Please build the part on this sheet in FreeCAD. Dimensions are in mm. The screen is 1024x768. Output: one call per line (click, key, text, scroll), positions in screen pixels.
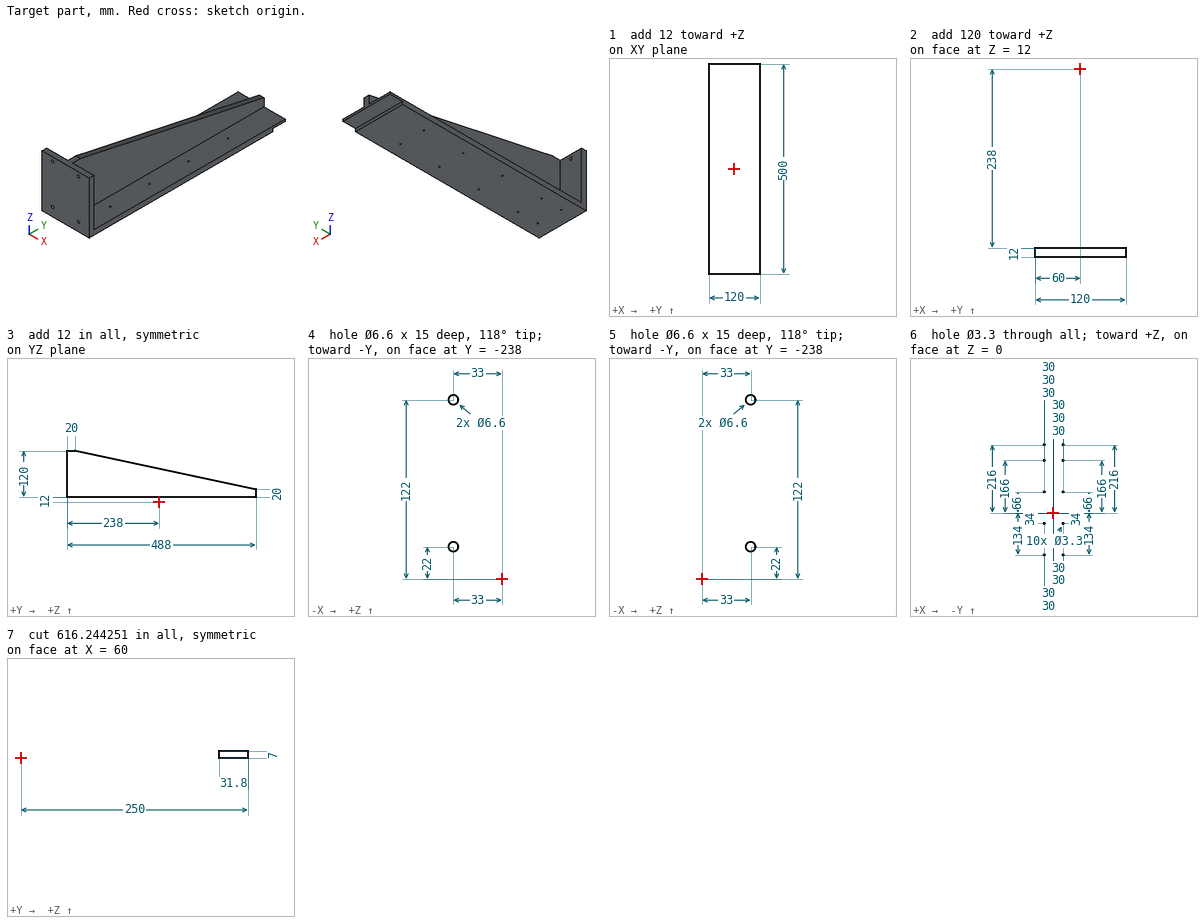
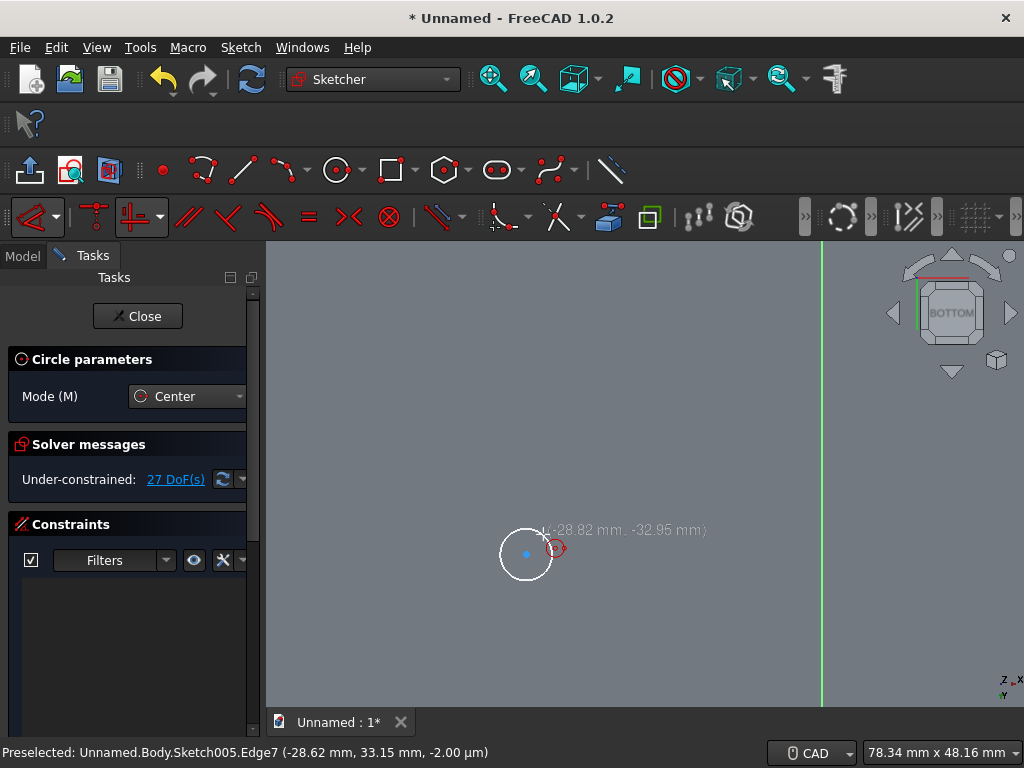
scroll(552, 539, down, 12)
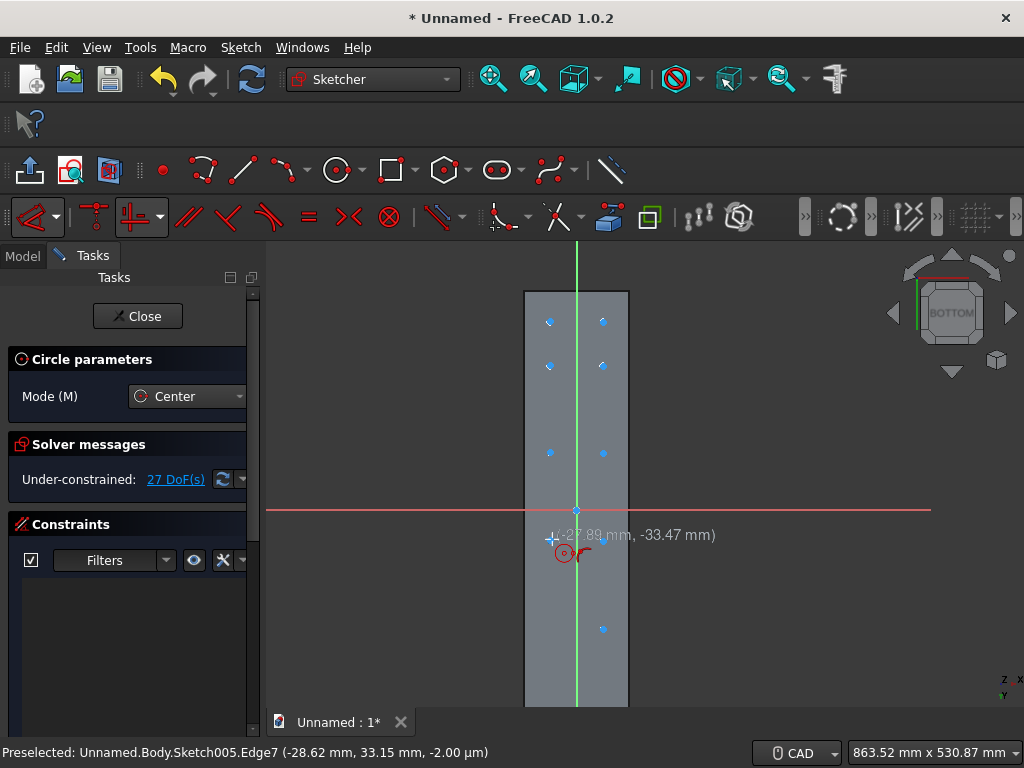
scroll(550, 628, up, 14)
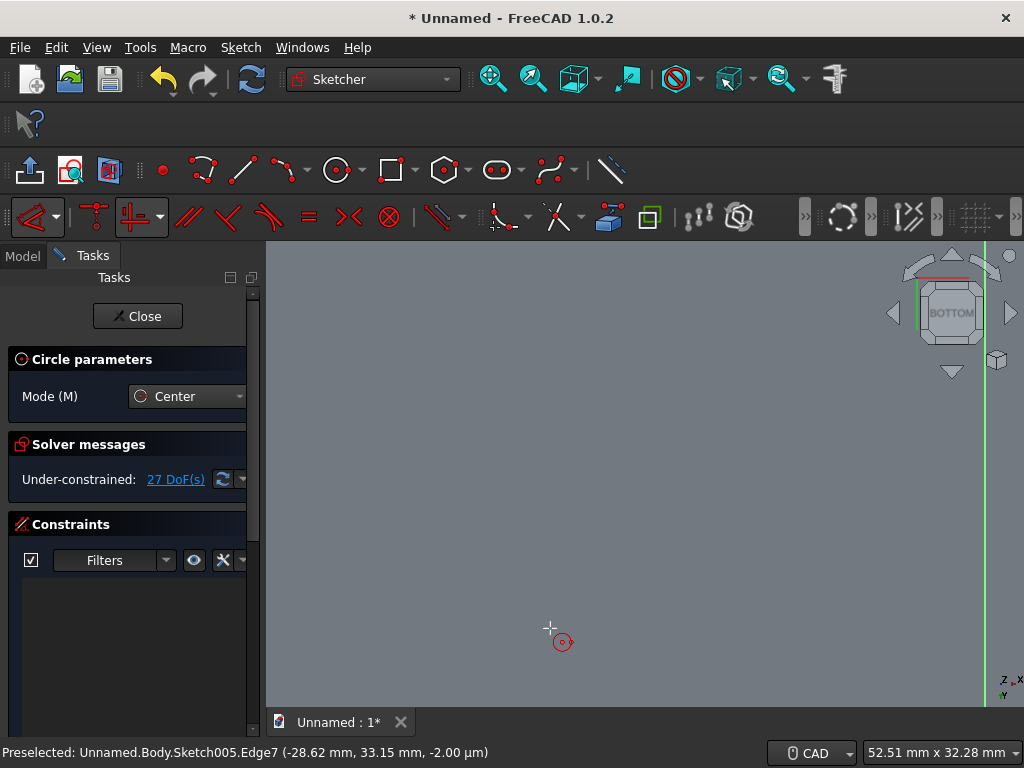
scroll(550, 629, down, 14)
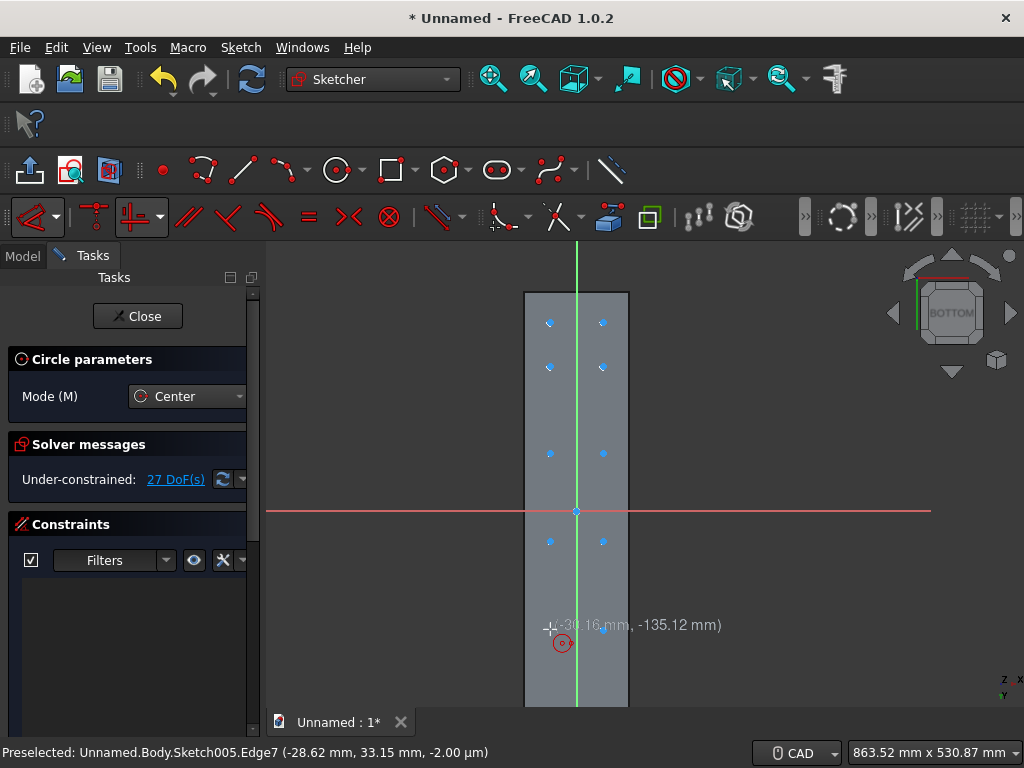
click(550, 629)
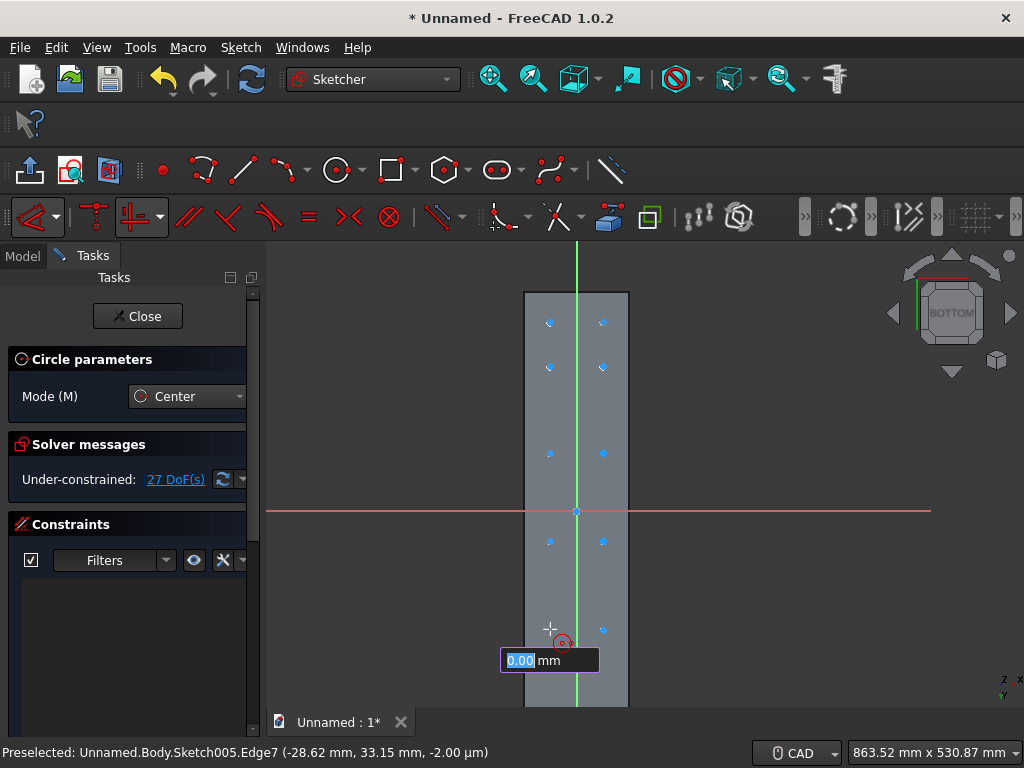
scroll(552, 628, up, 12)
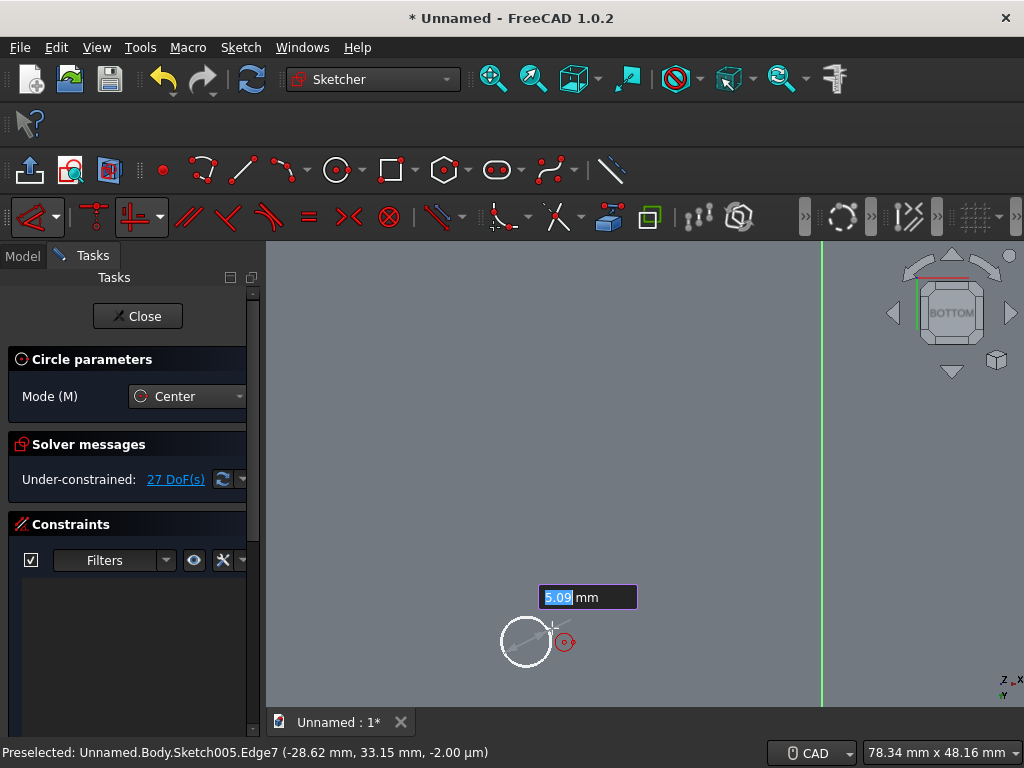
click(543, 618)
key(Escape)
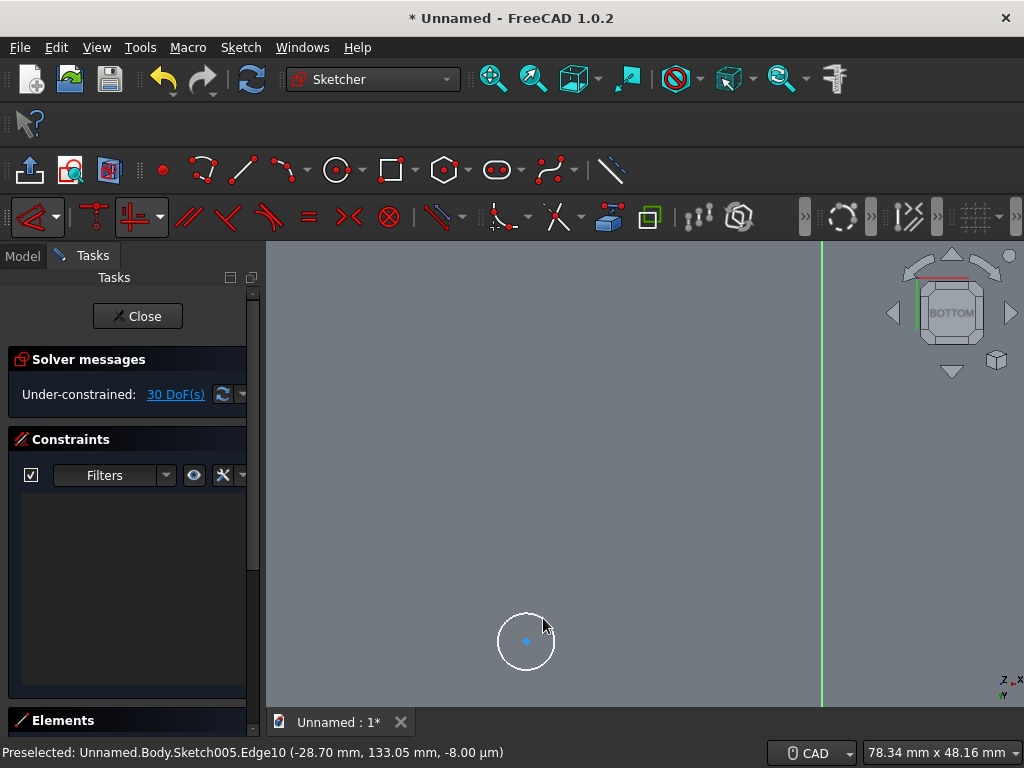
scroll(552, 627, down, 12)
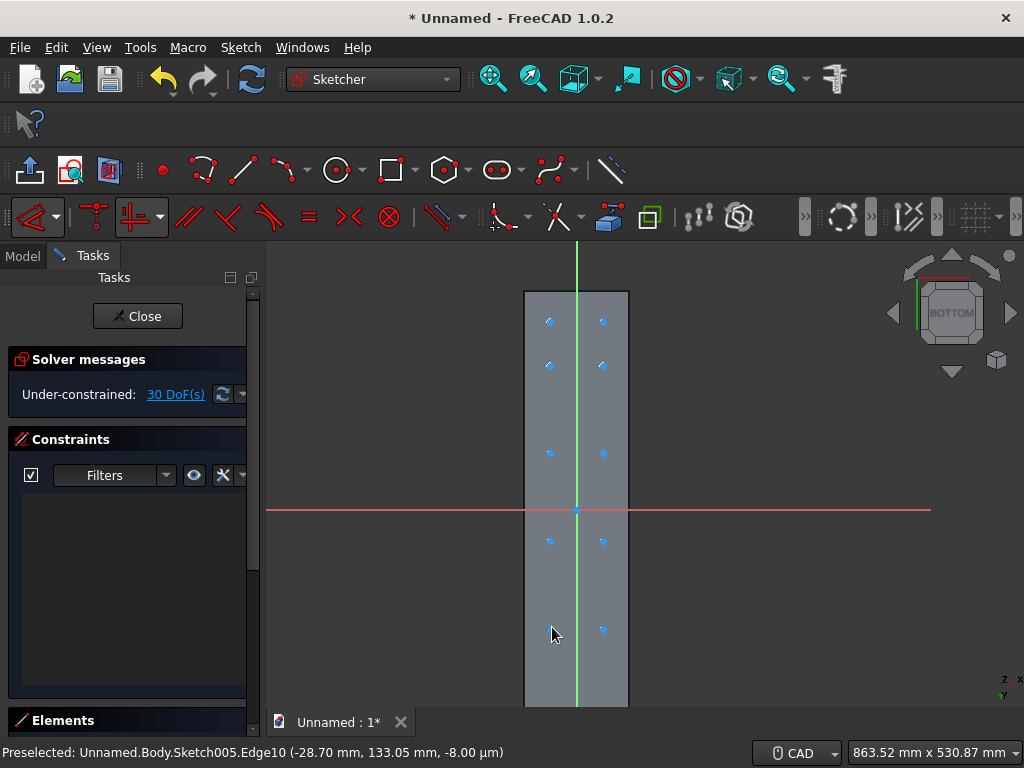
scroll(605, 540, up, 10)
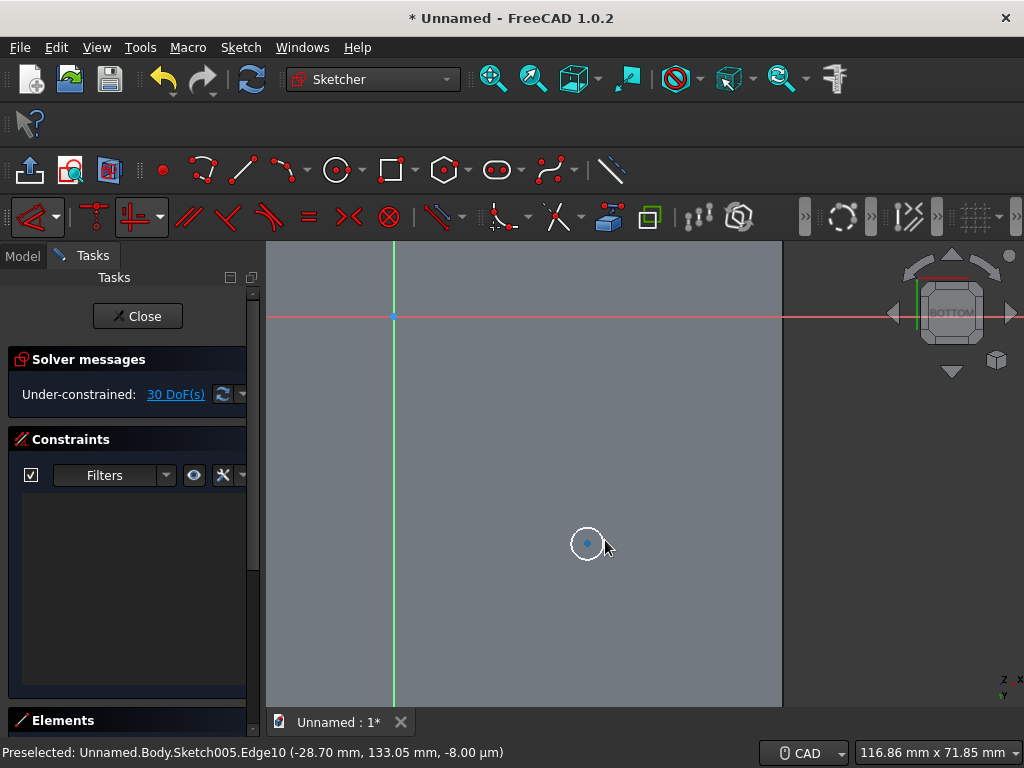
click(599, 532)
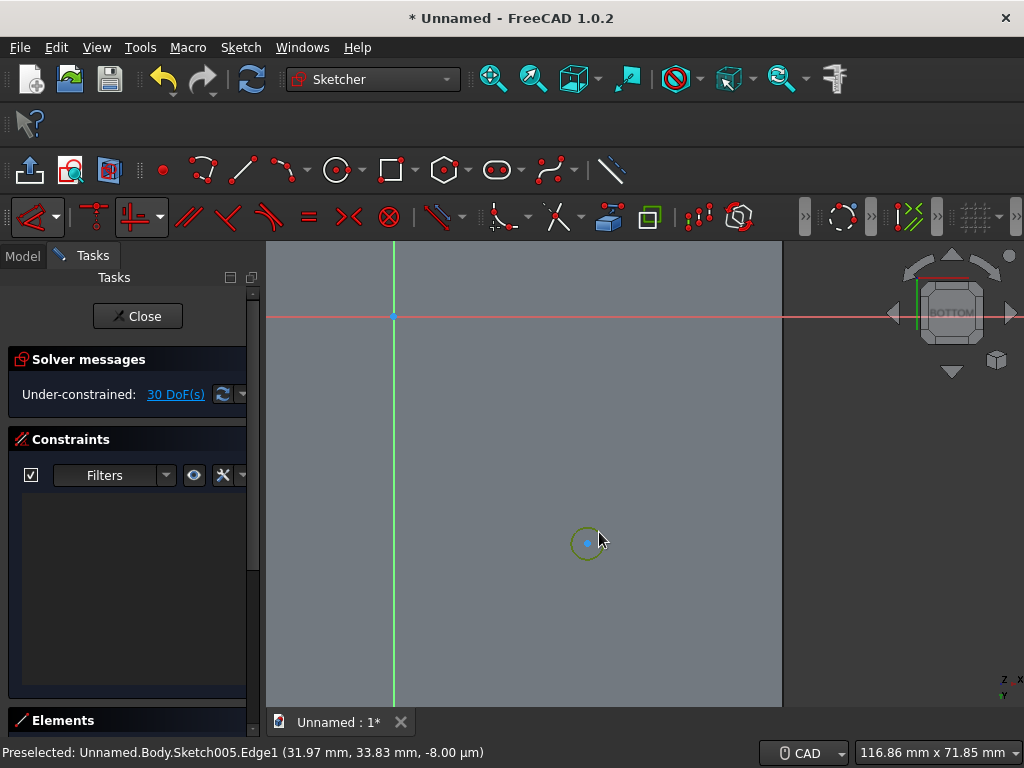
scroll(605, 540, down, 10)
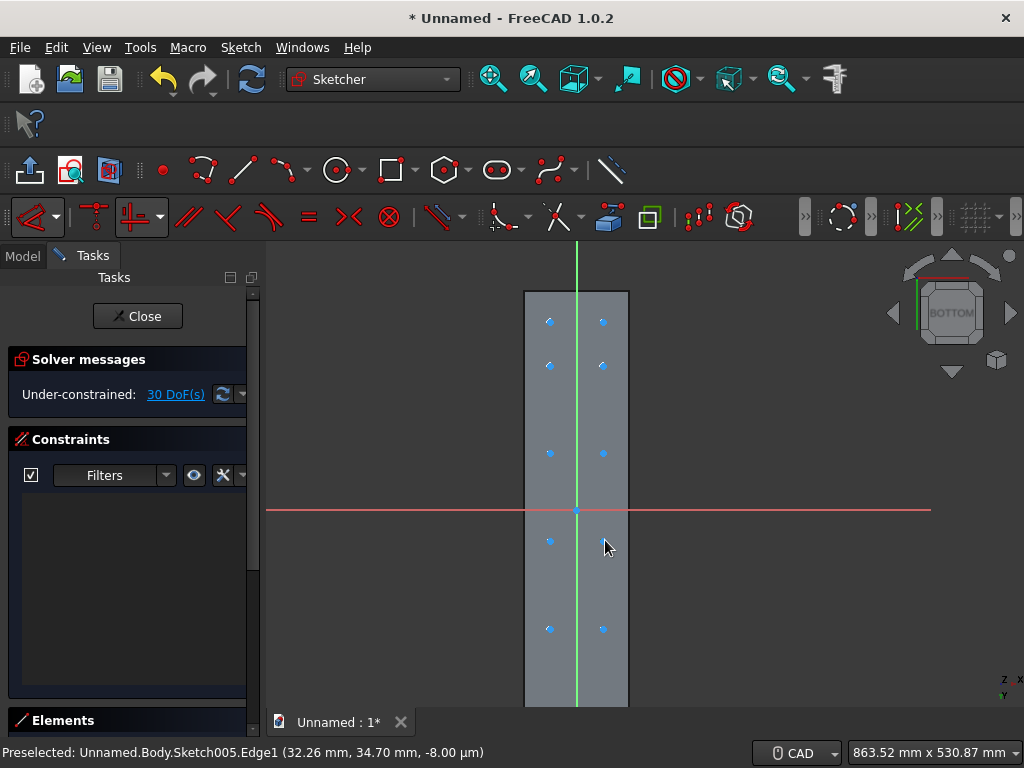
scroll(605, 627, up, 9)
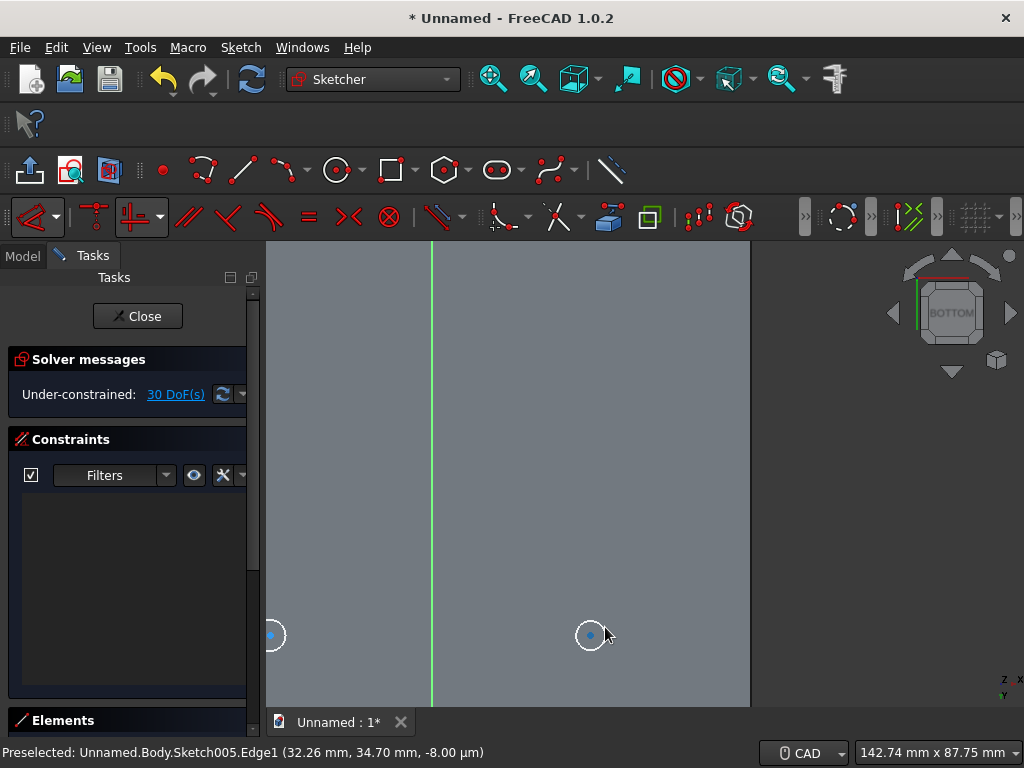
click(601, 625)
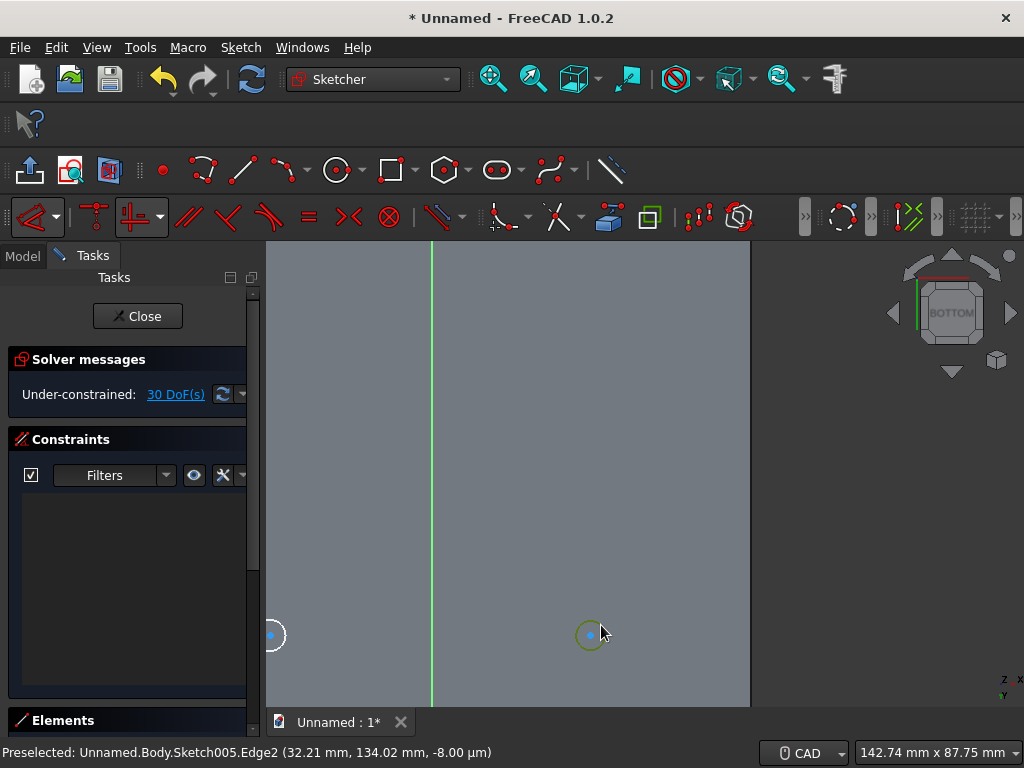
scroll(605, 627, down, 9)